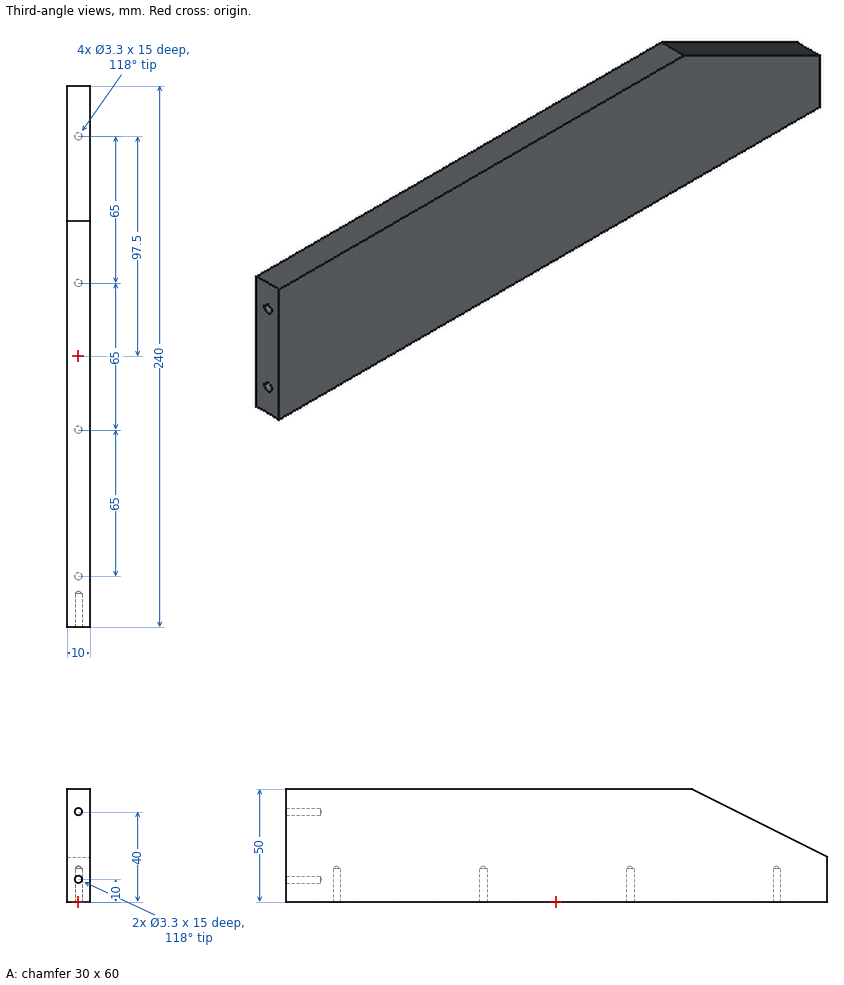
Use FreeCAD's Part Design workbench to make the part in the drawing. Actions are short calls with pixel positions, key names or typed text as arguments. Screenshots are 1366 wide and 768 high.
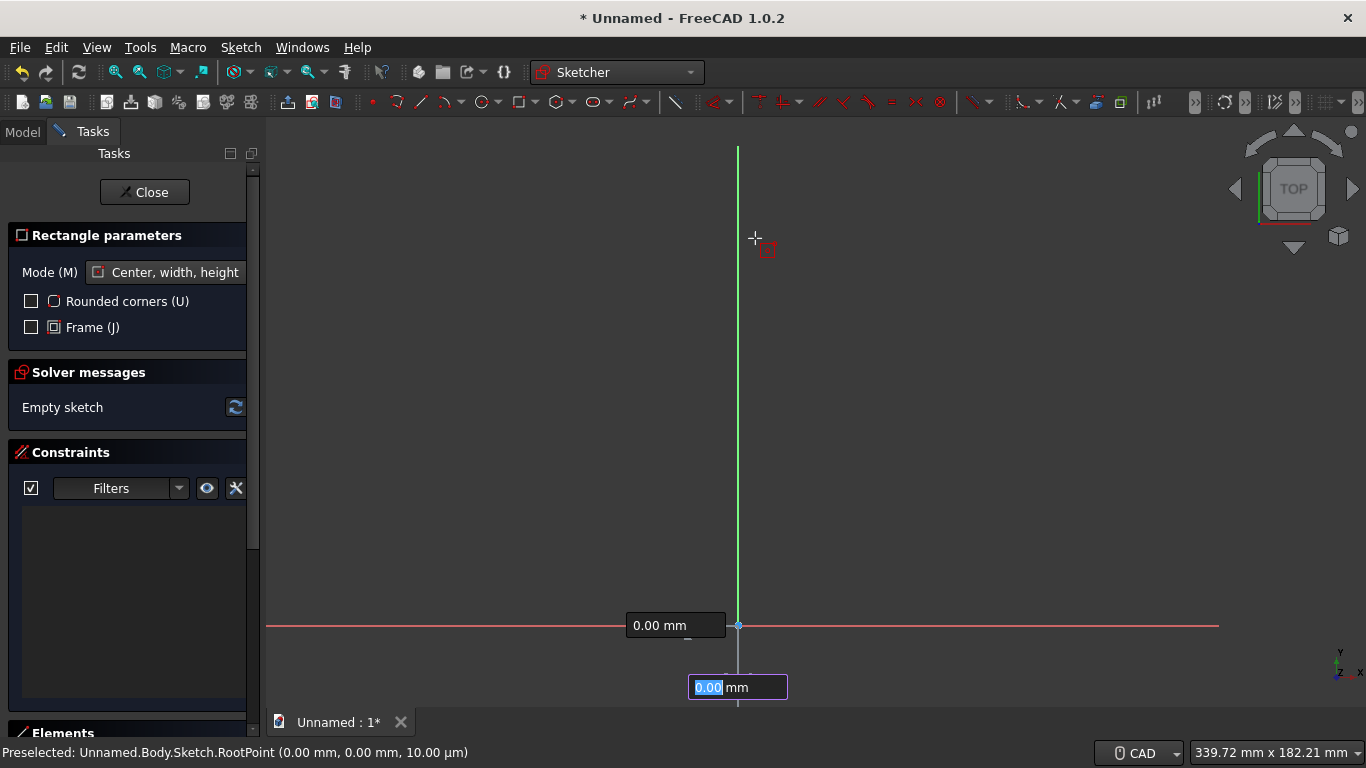
click(755, 237)
key(Escape)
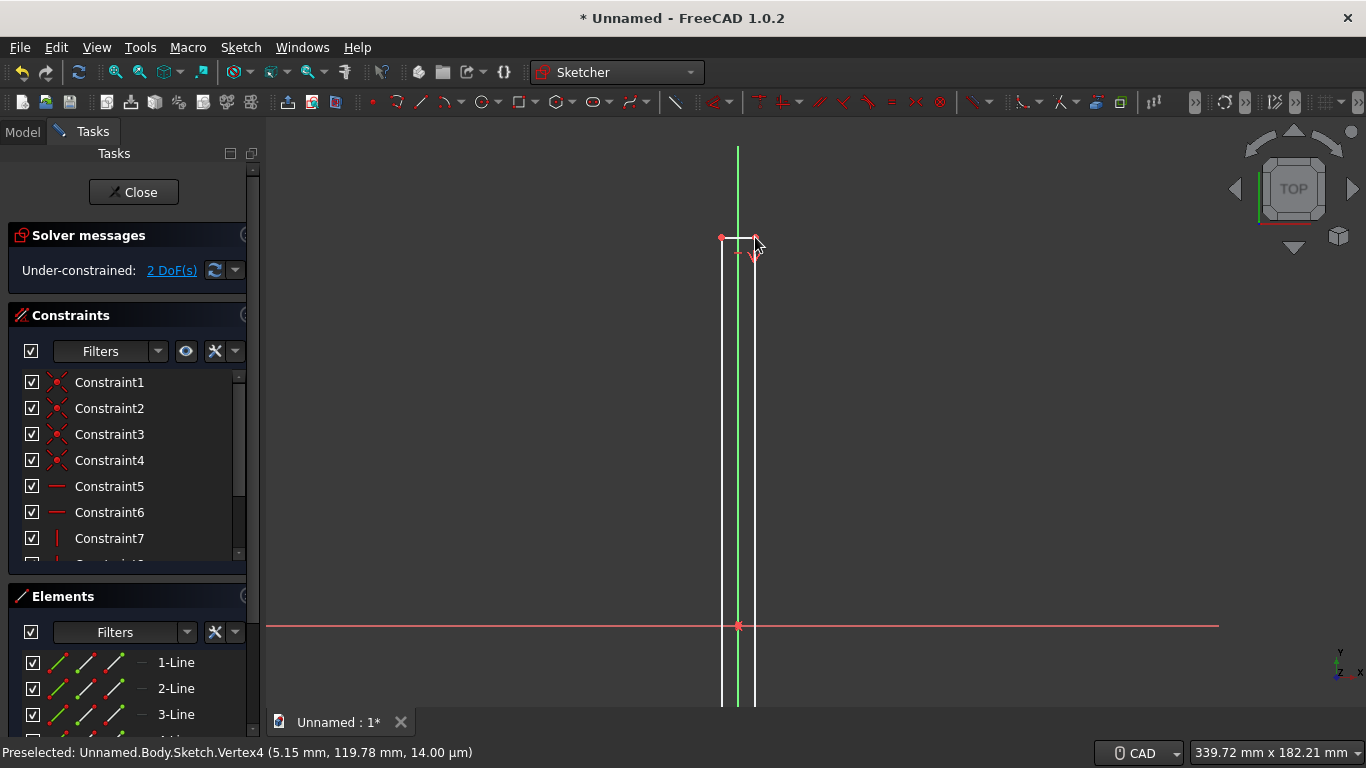
key(d)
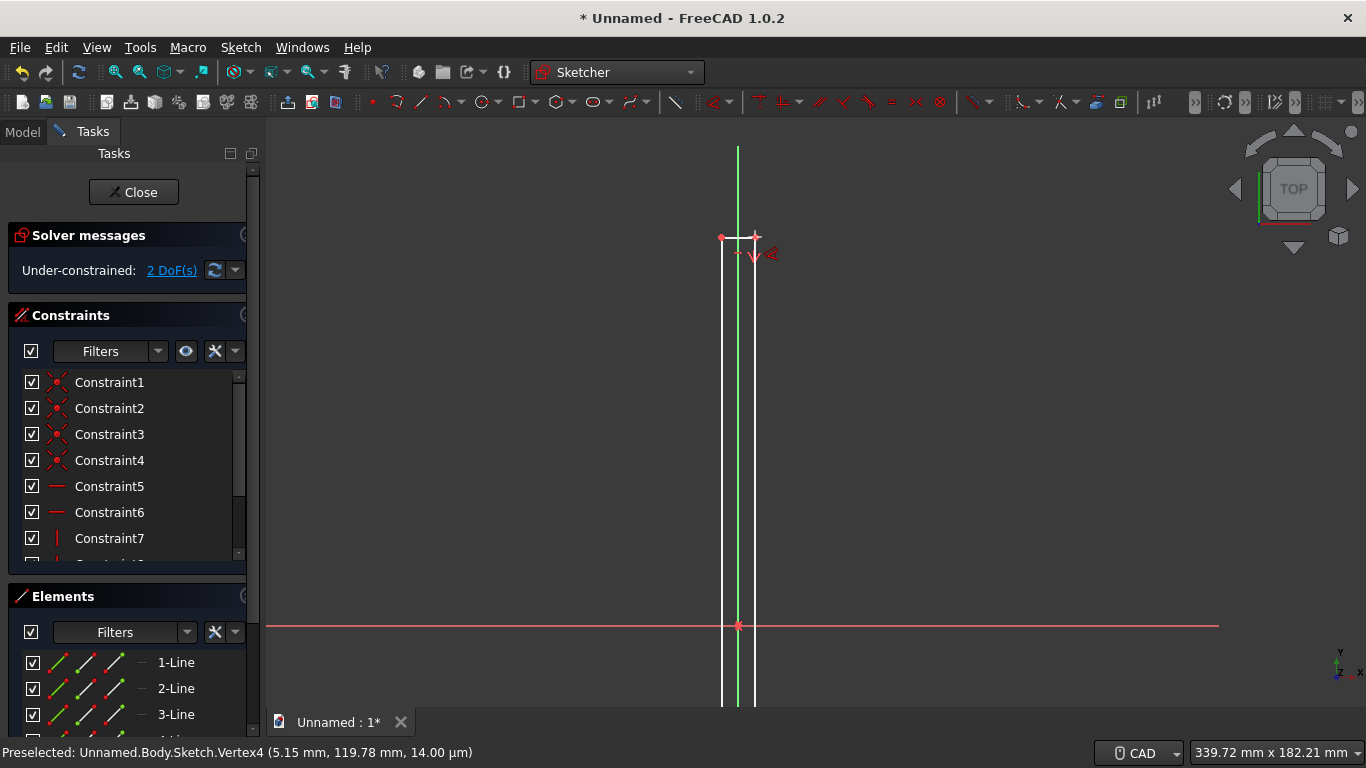
scroll(755, 238, down, 4)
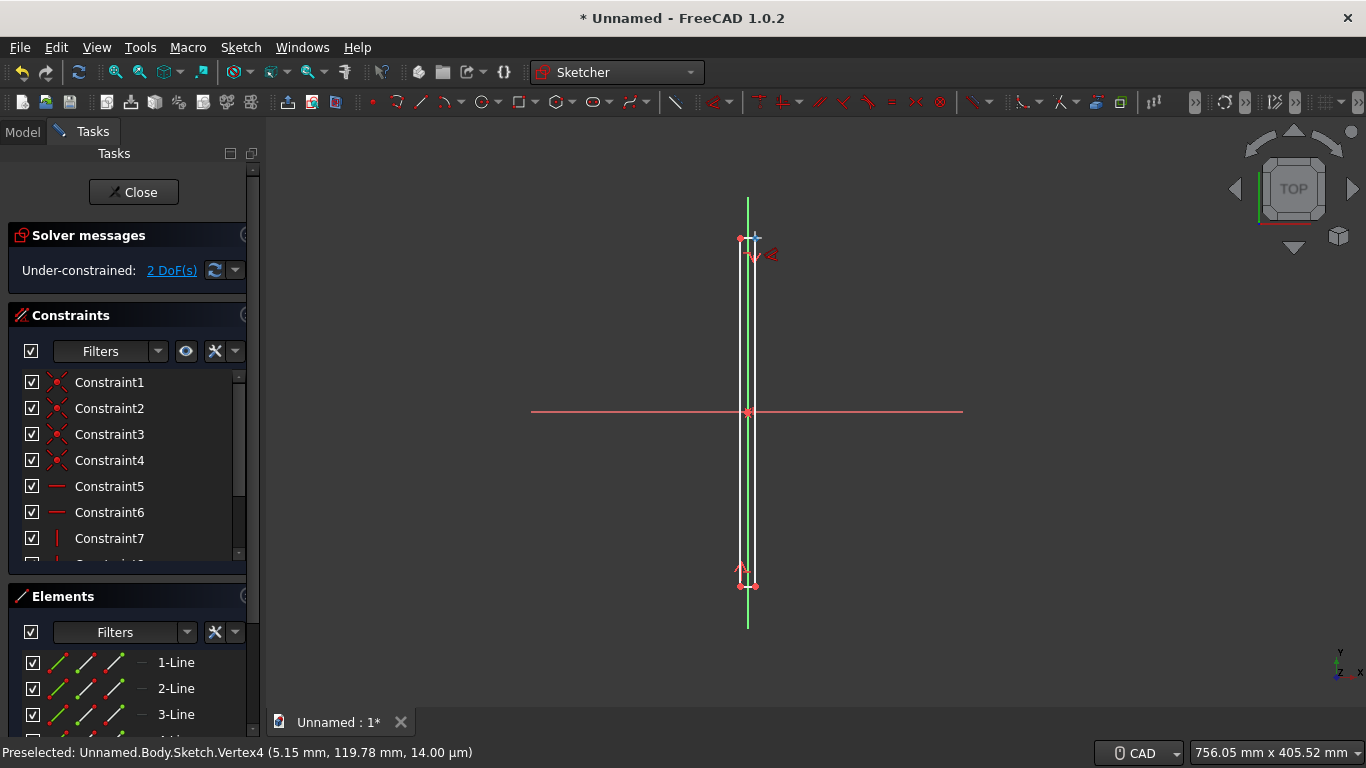
scroll(746, 587, up, 6)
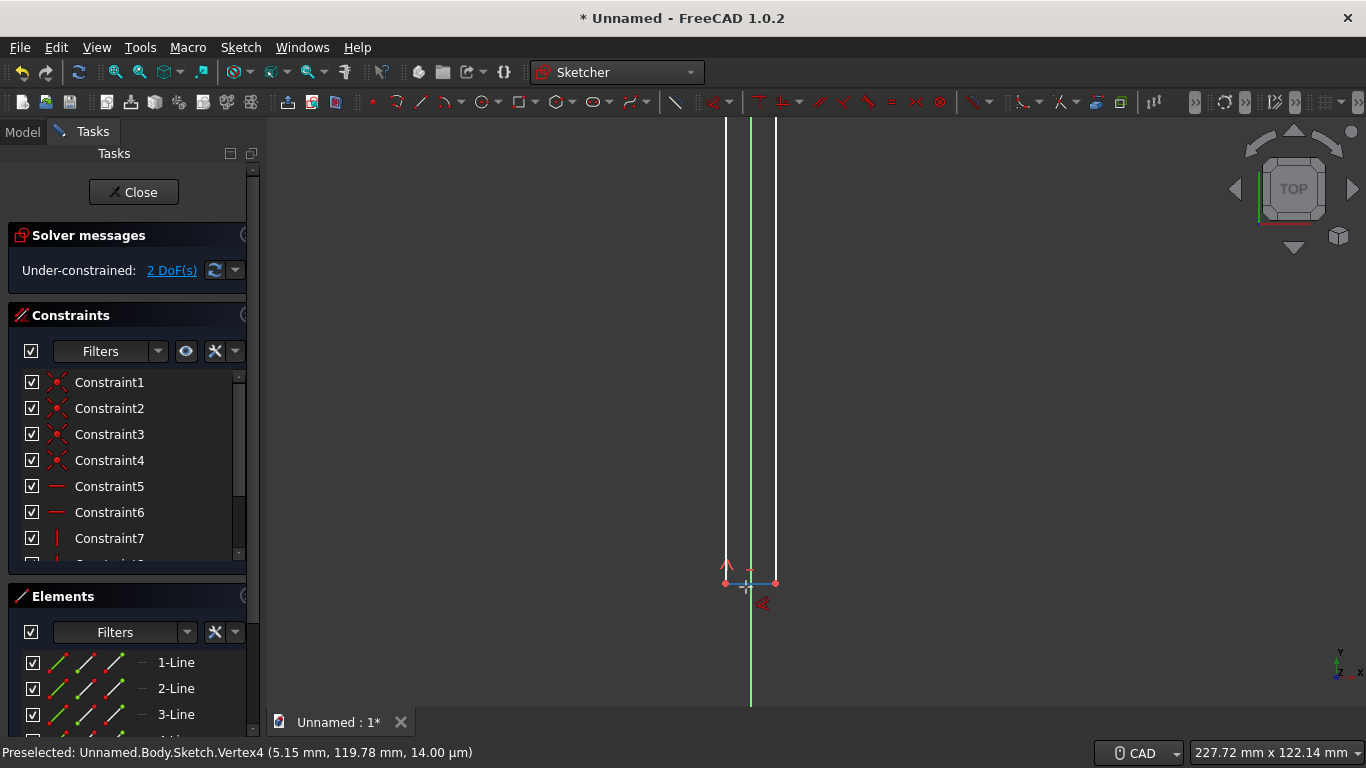
click(746, 584)
click(733, 618)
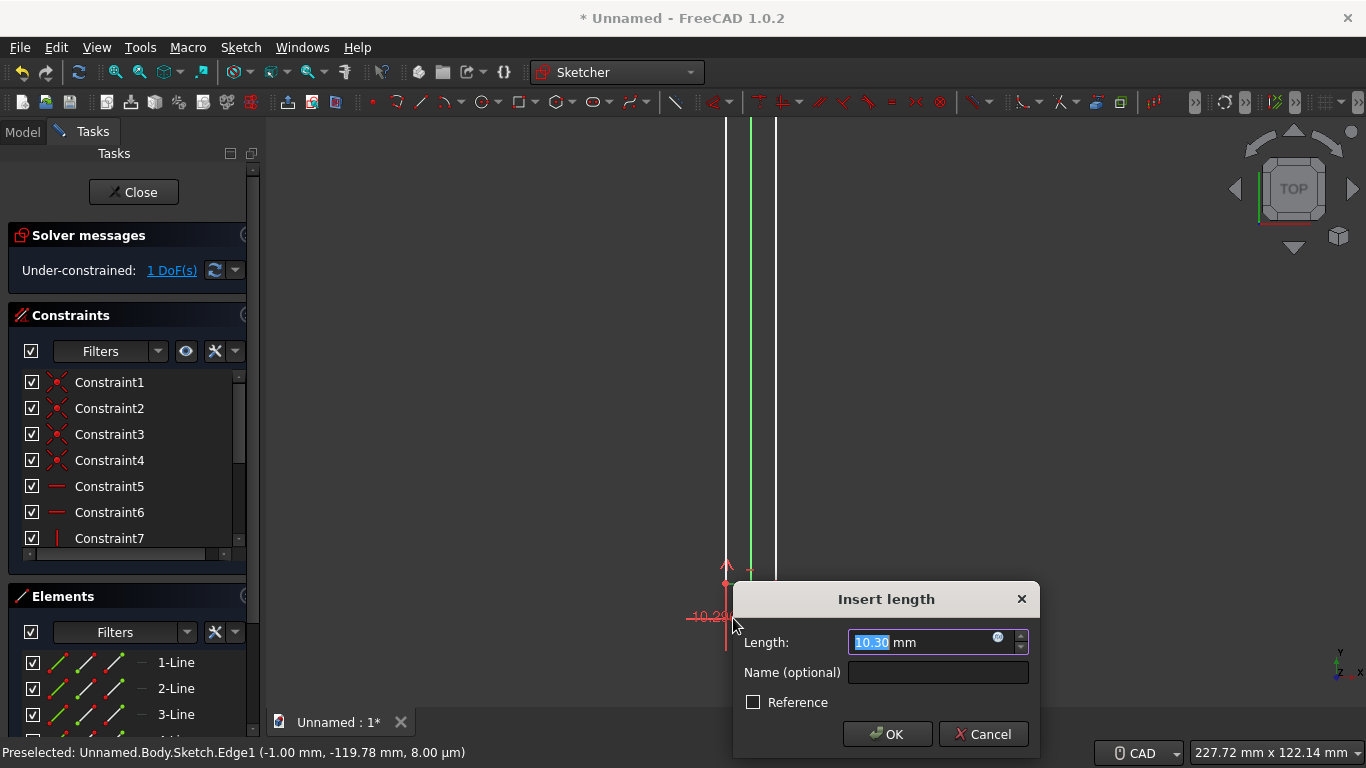
text(10)
key(Return)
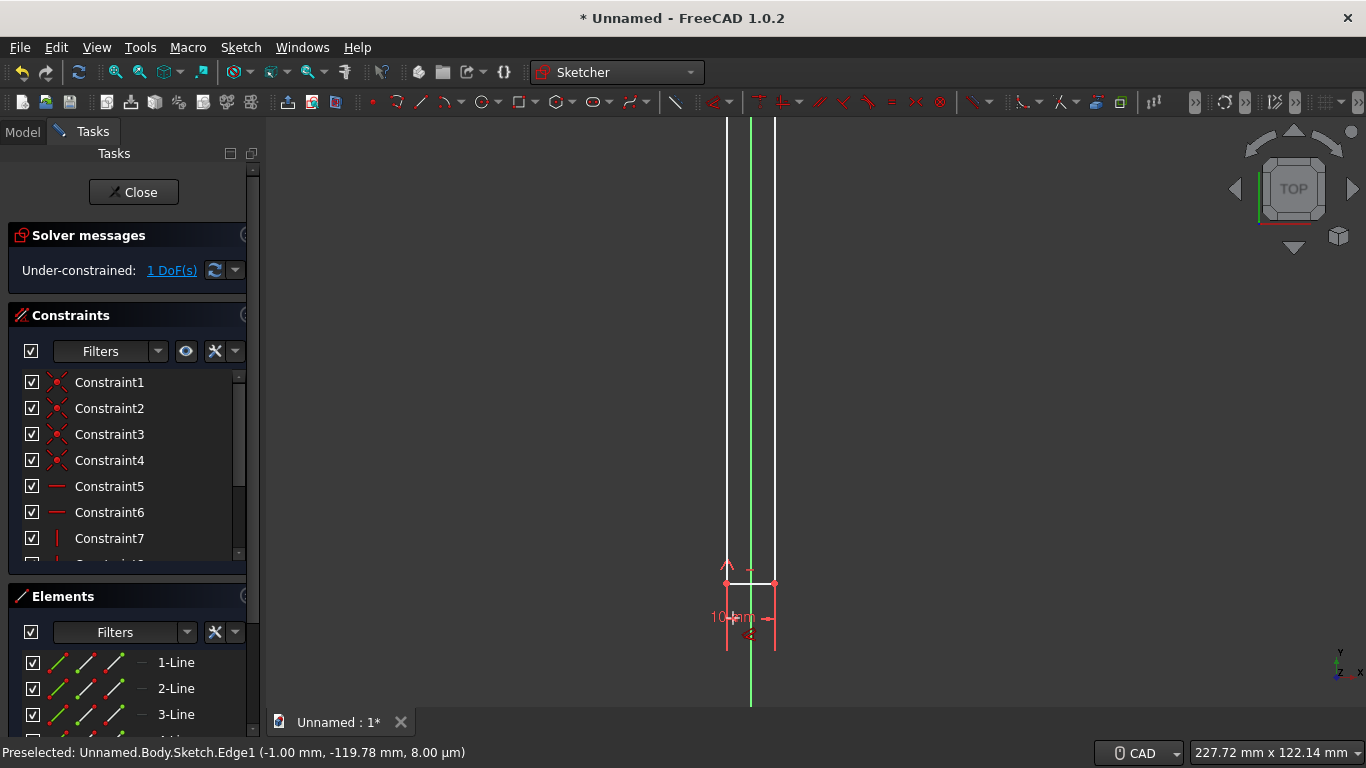
click(775, 237)
click(809, 364)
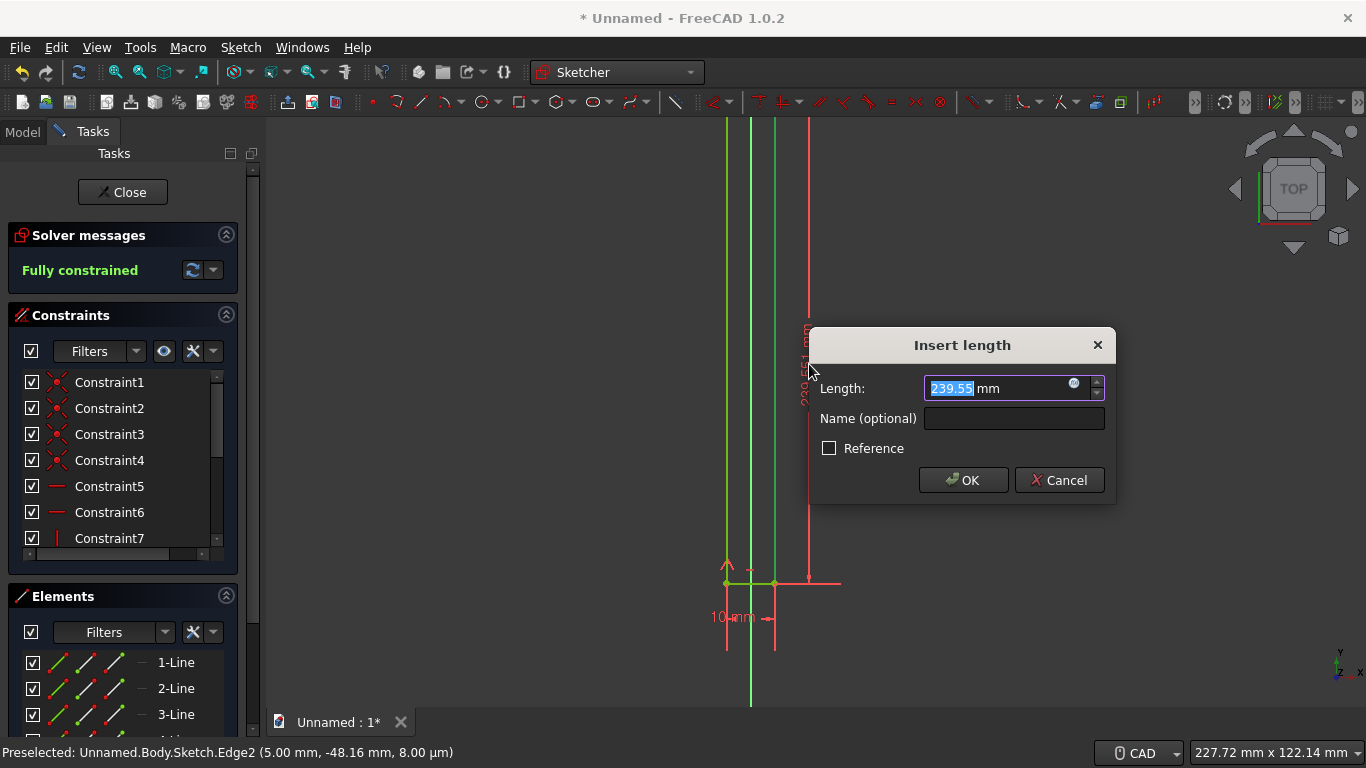
text(240)
key(Return)
key(Escape)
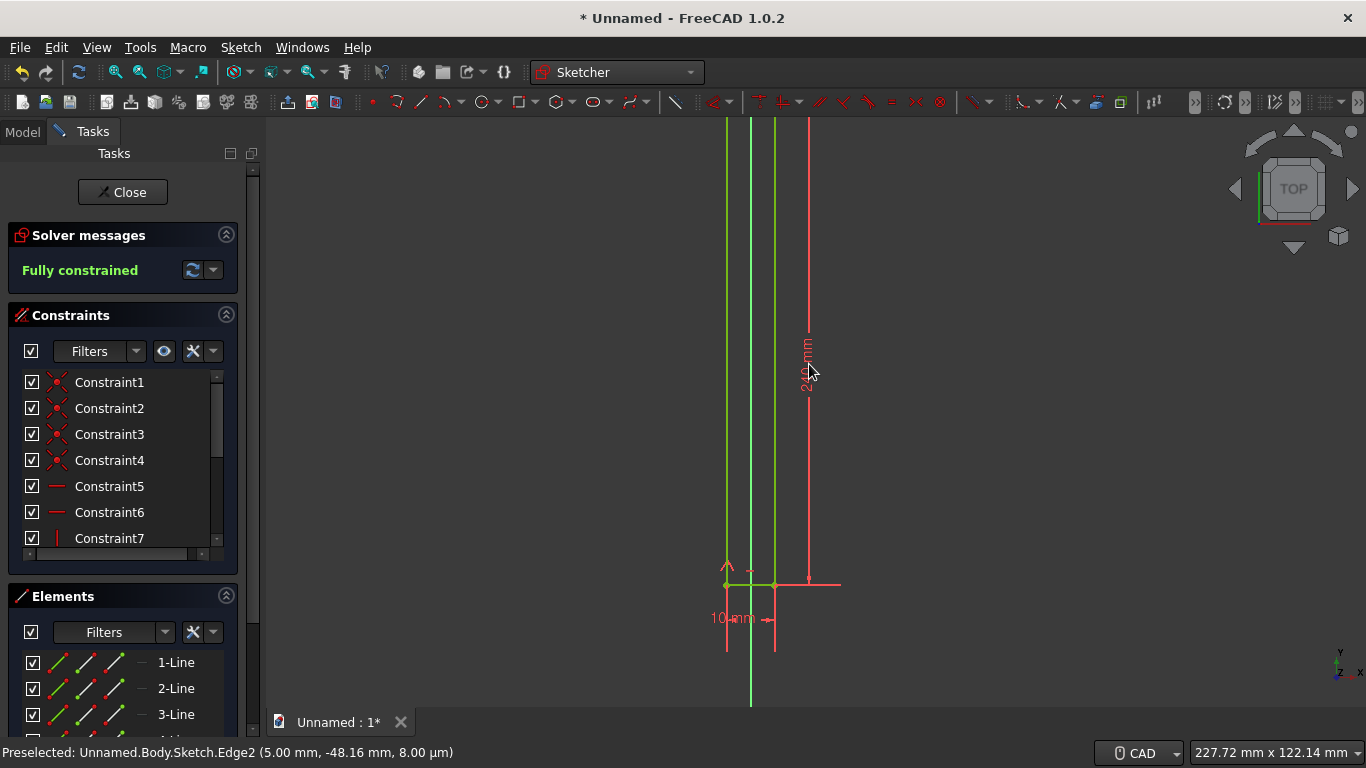
click(123, 192)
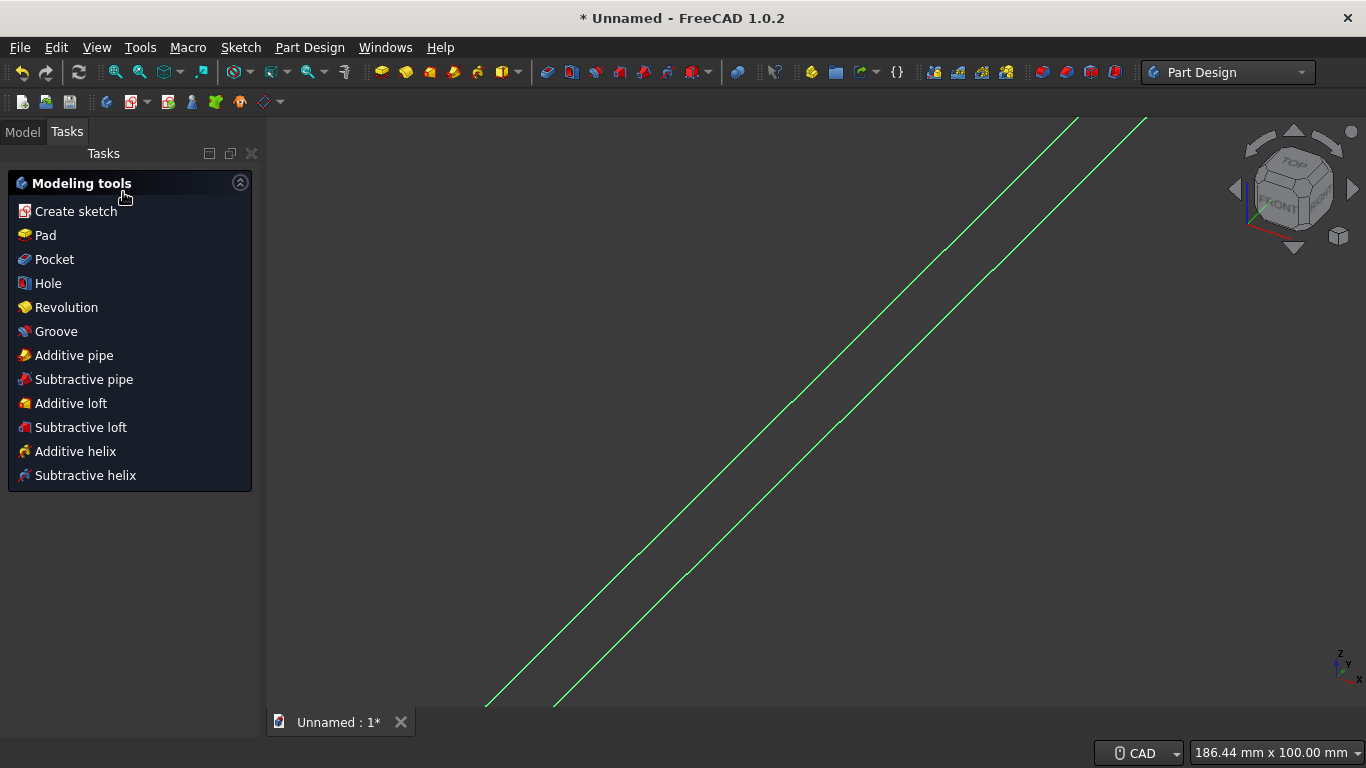
click(382, 72)